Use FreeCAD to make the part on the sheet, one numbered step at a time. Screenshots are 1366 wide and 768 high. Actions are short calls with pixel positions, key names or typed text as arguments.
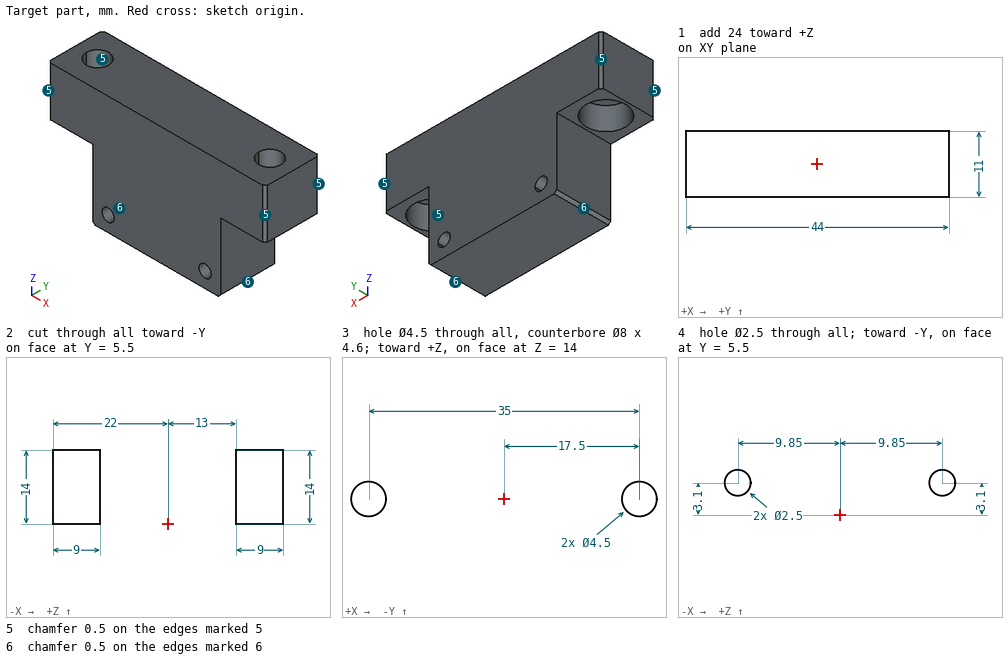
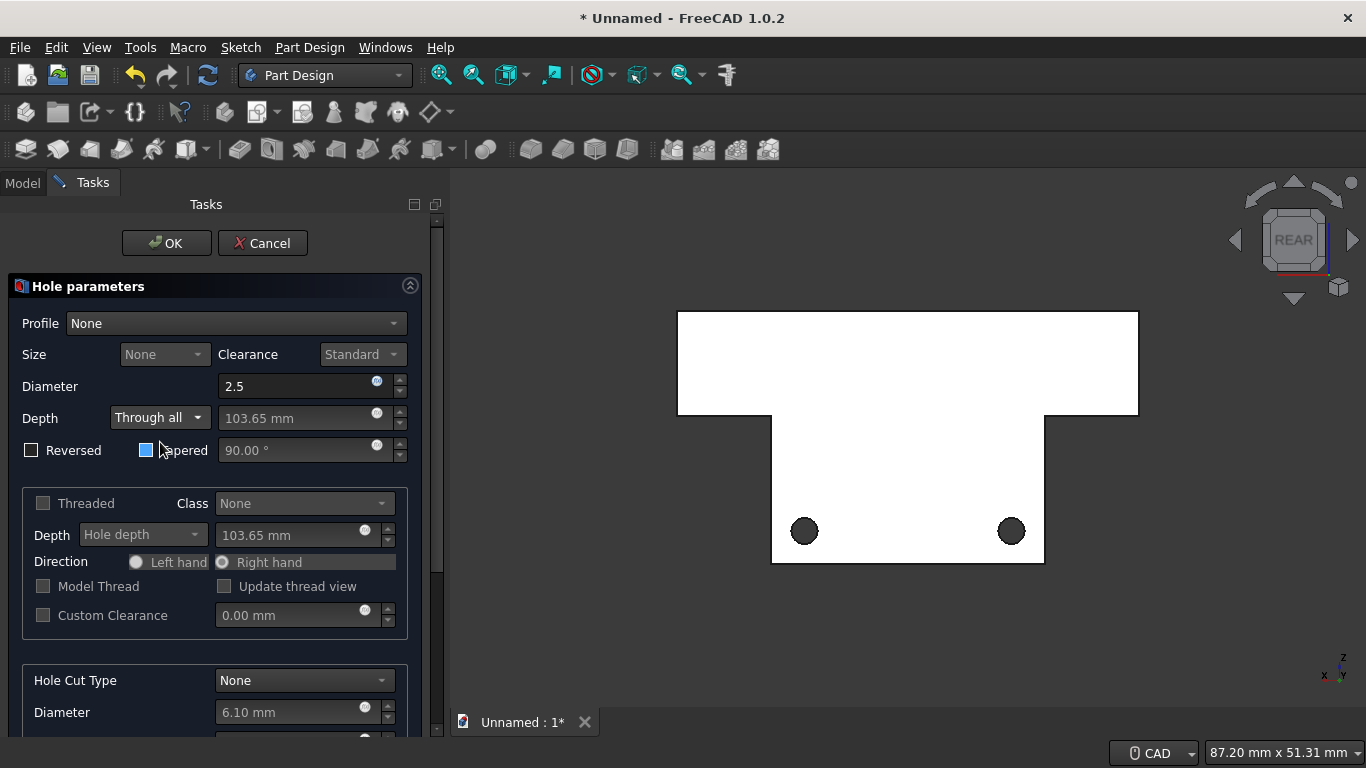
click(167, 243)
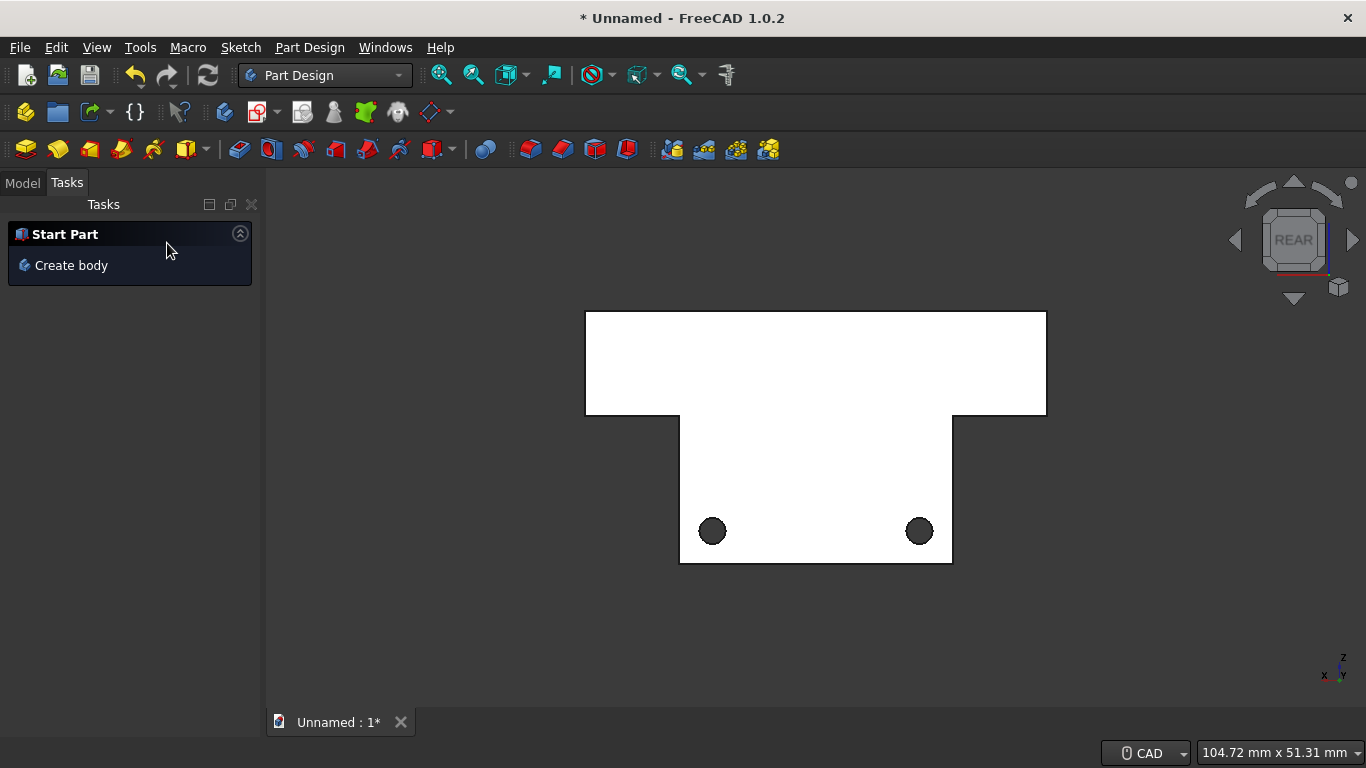
click(1047, 363)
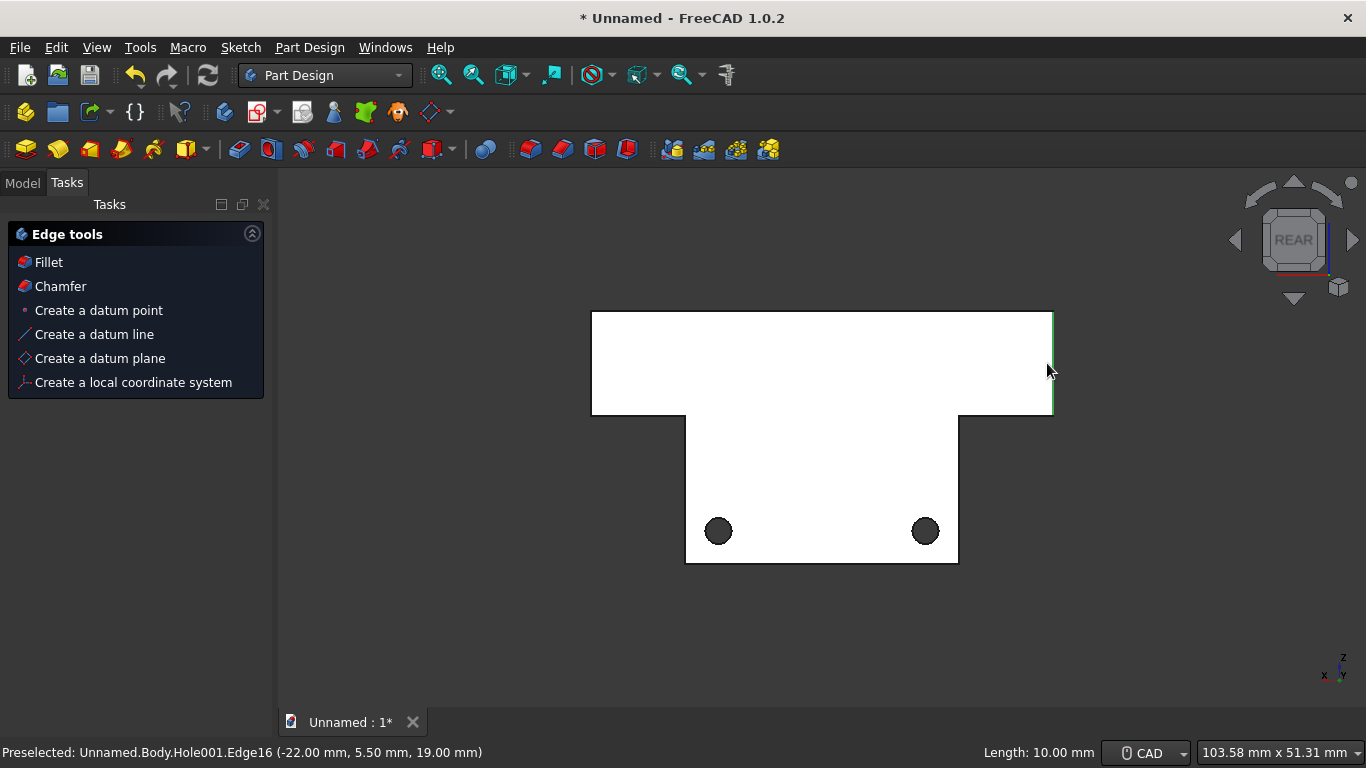
key(0)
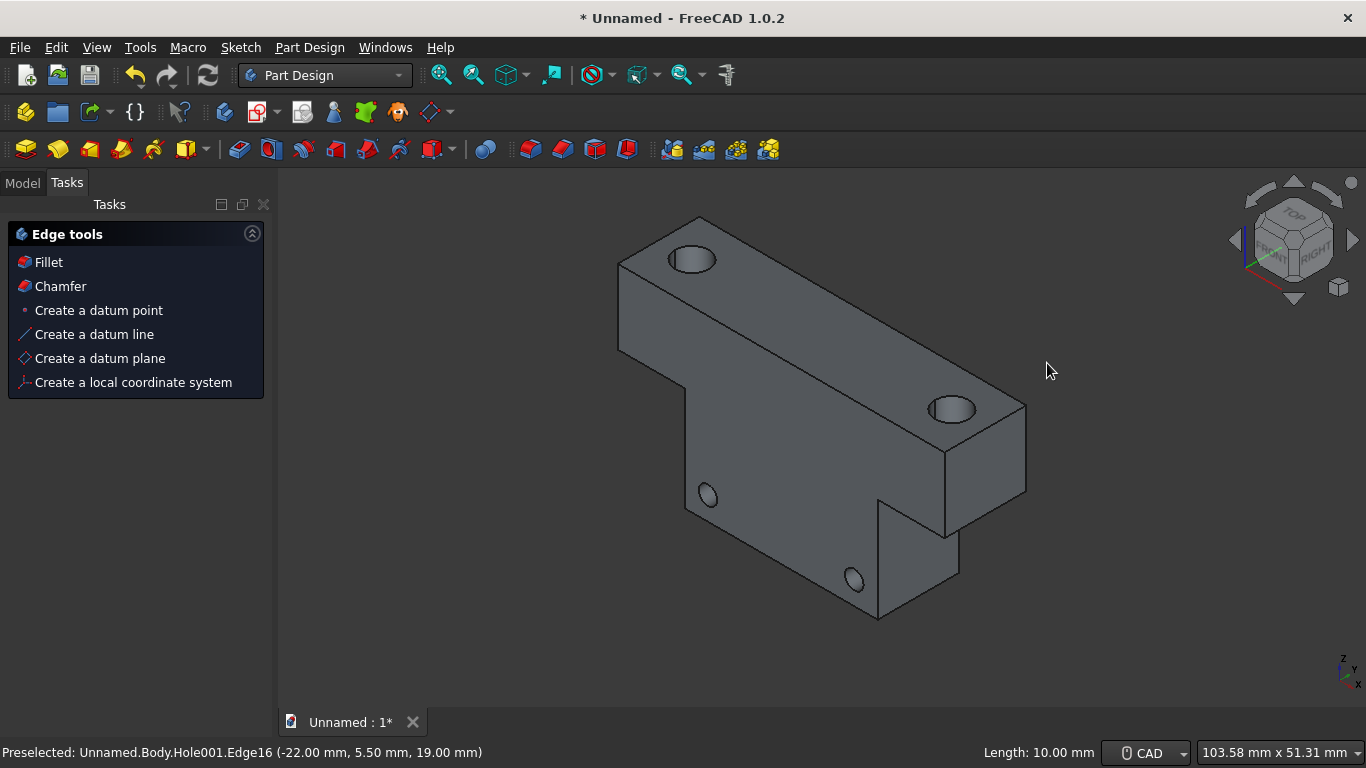
click(945, 494, ctrl)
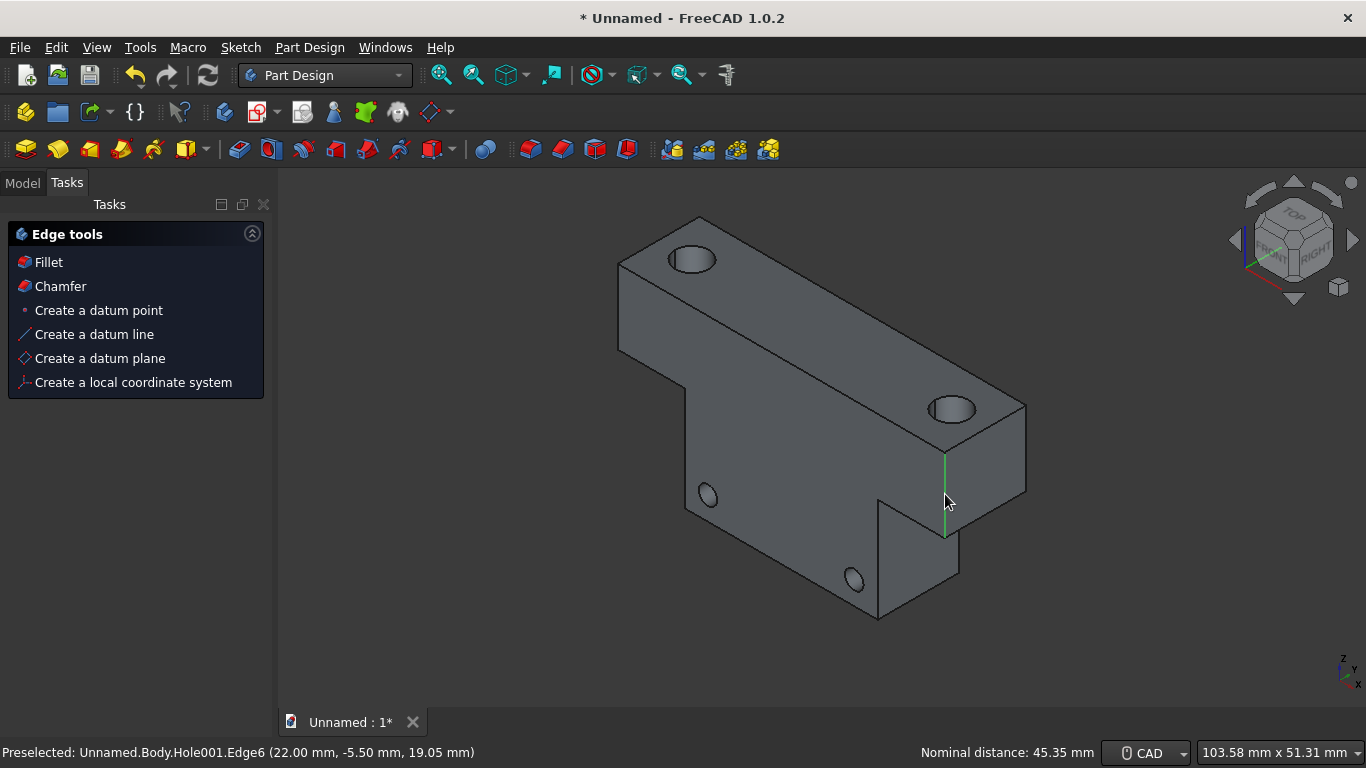
key(2)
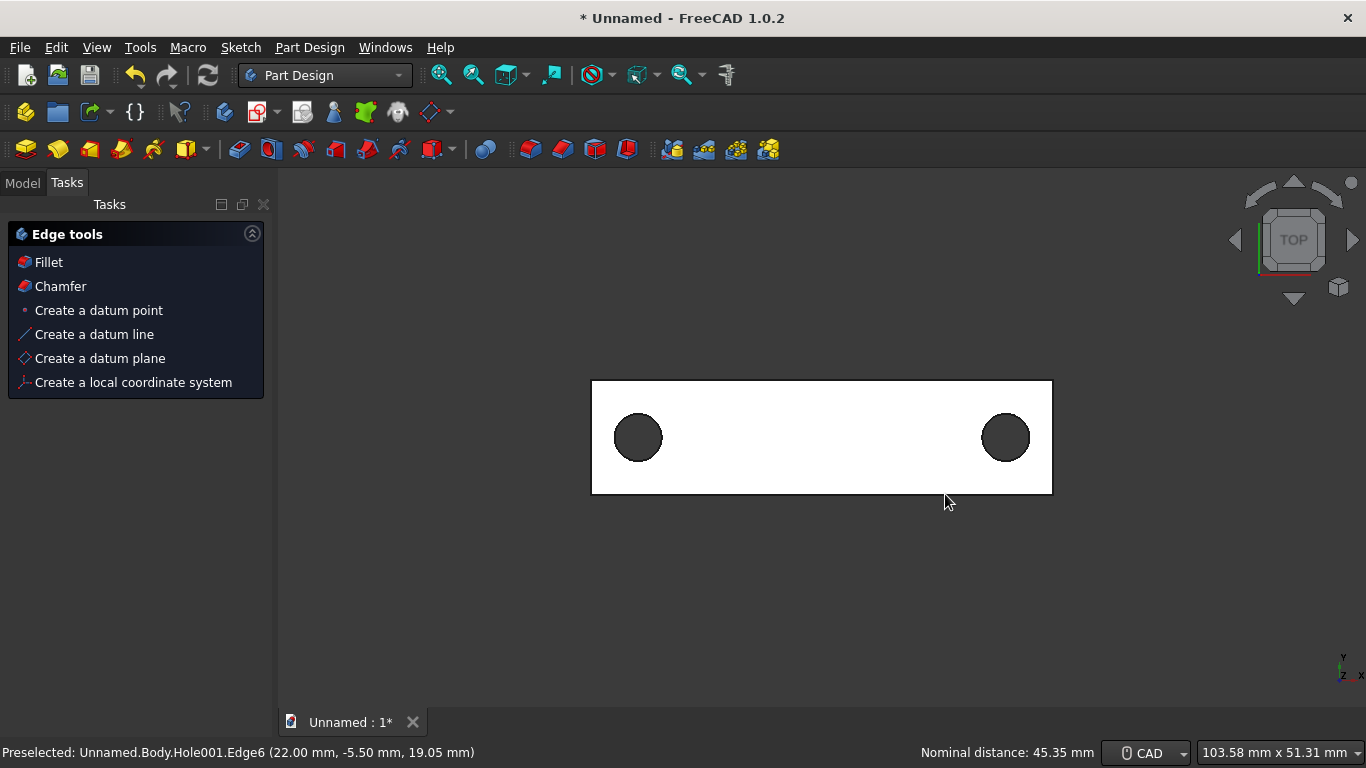
click(442, 76)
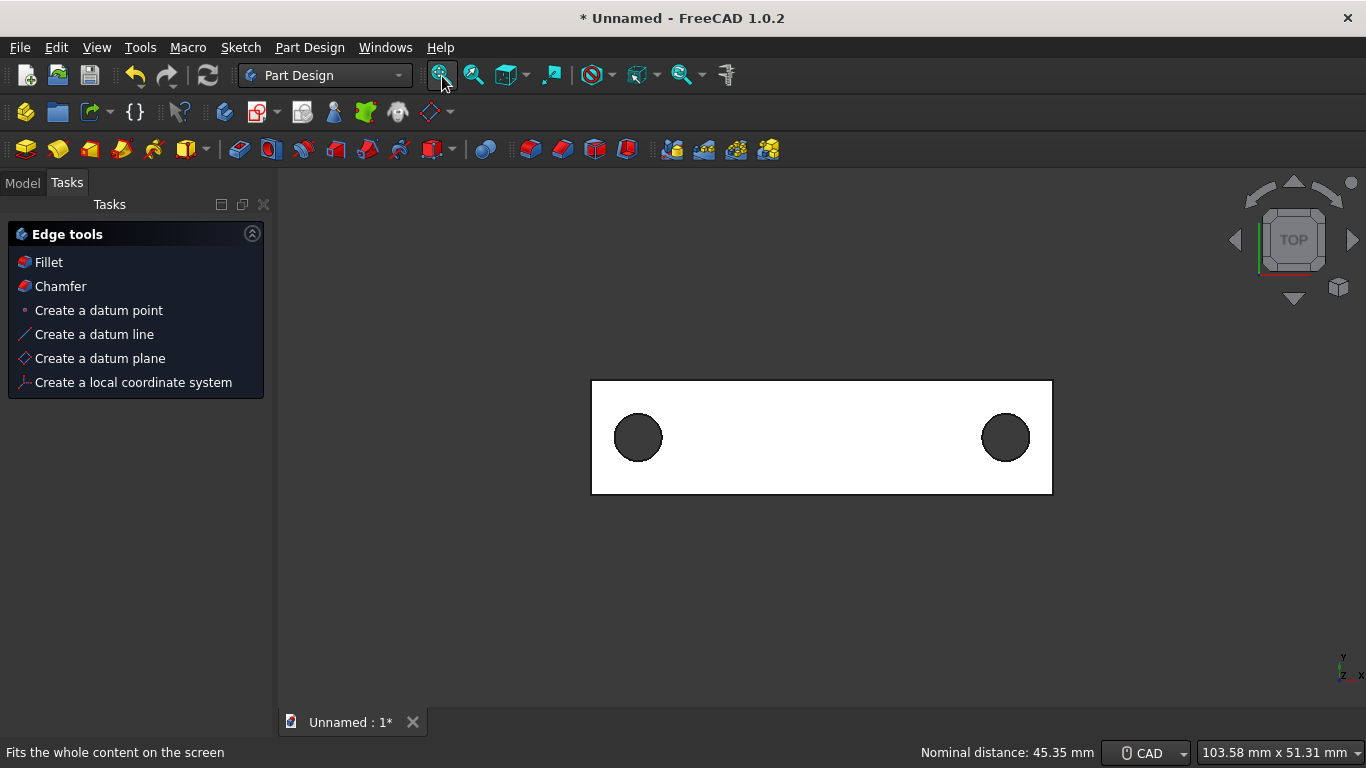
key(1)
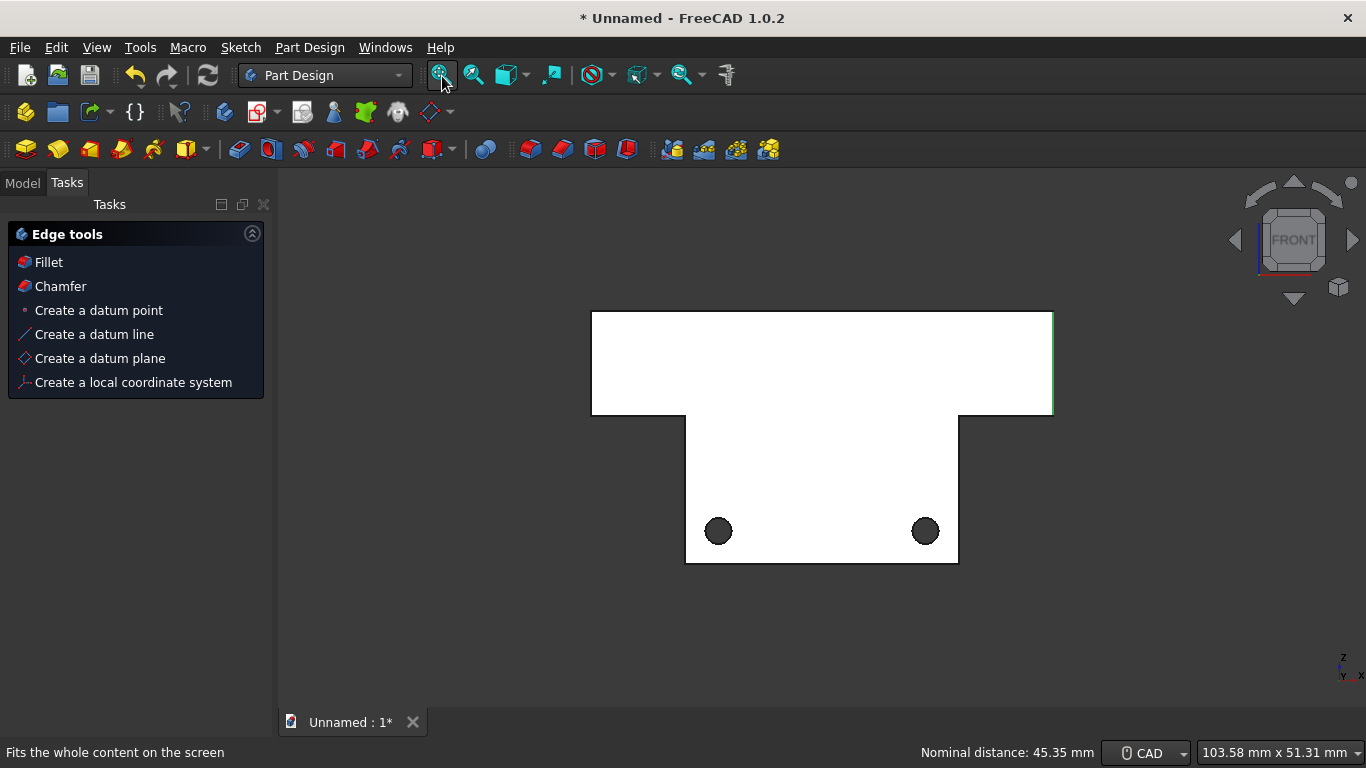
click(591, 363, ctrl)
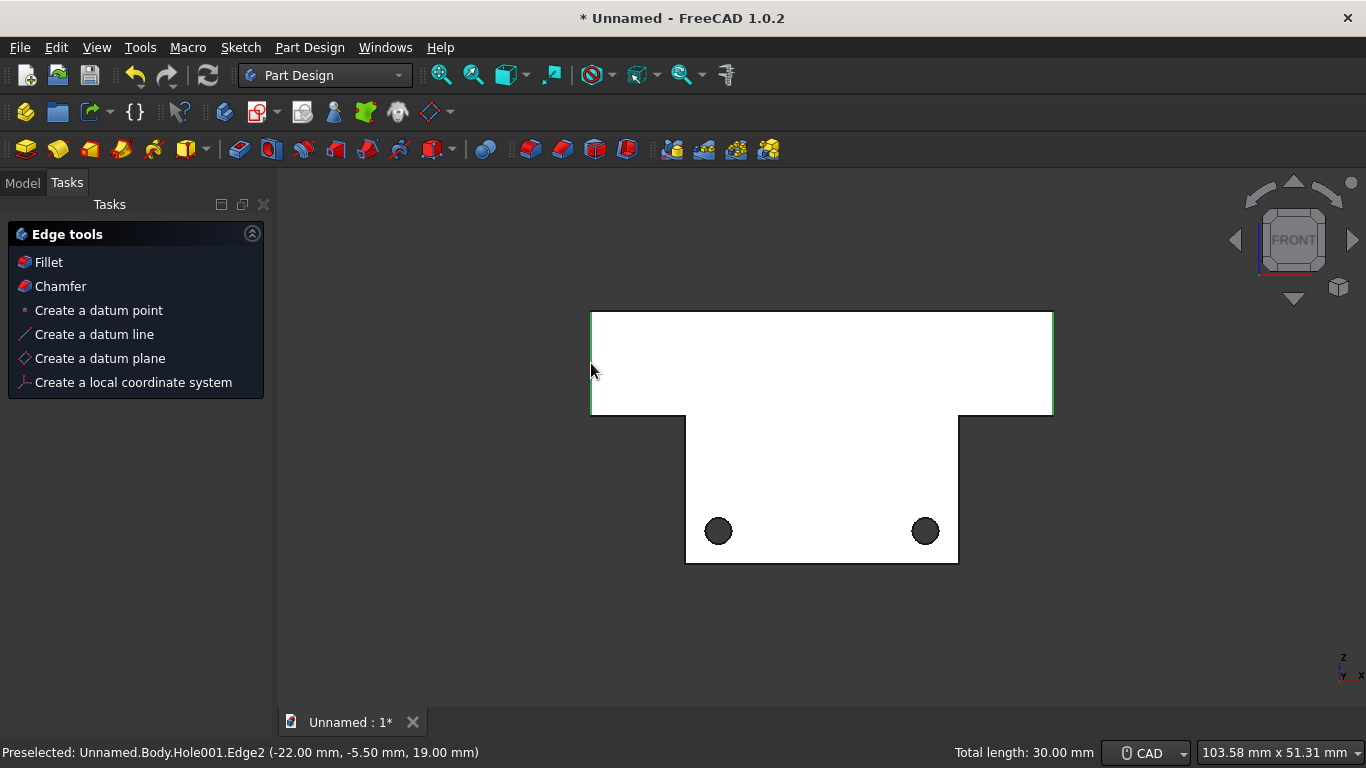
key(3)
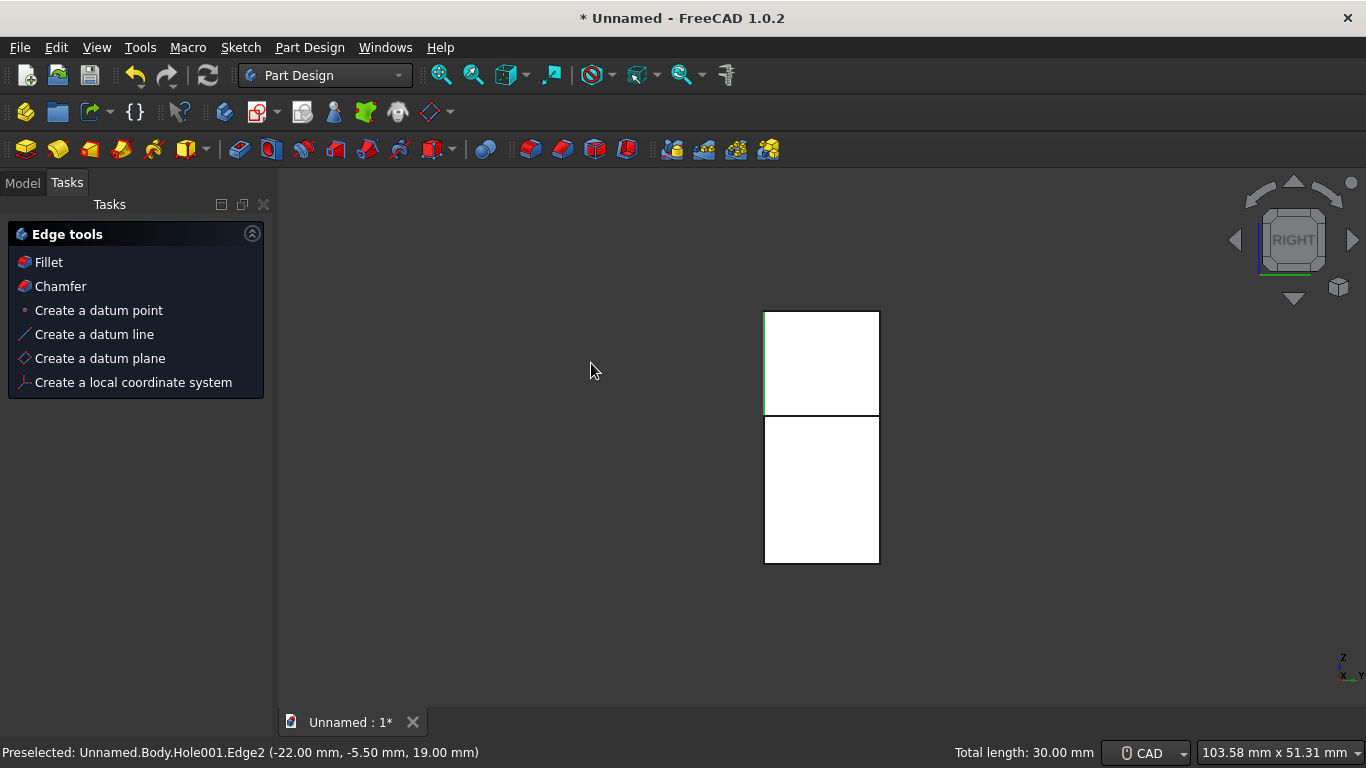
click(880, 363, ctrl)